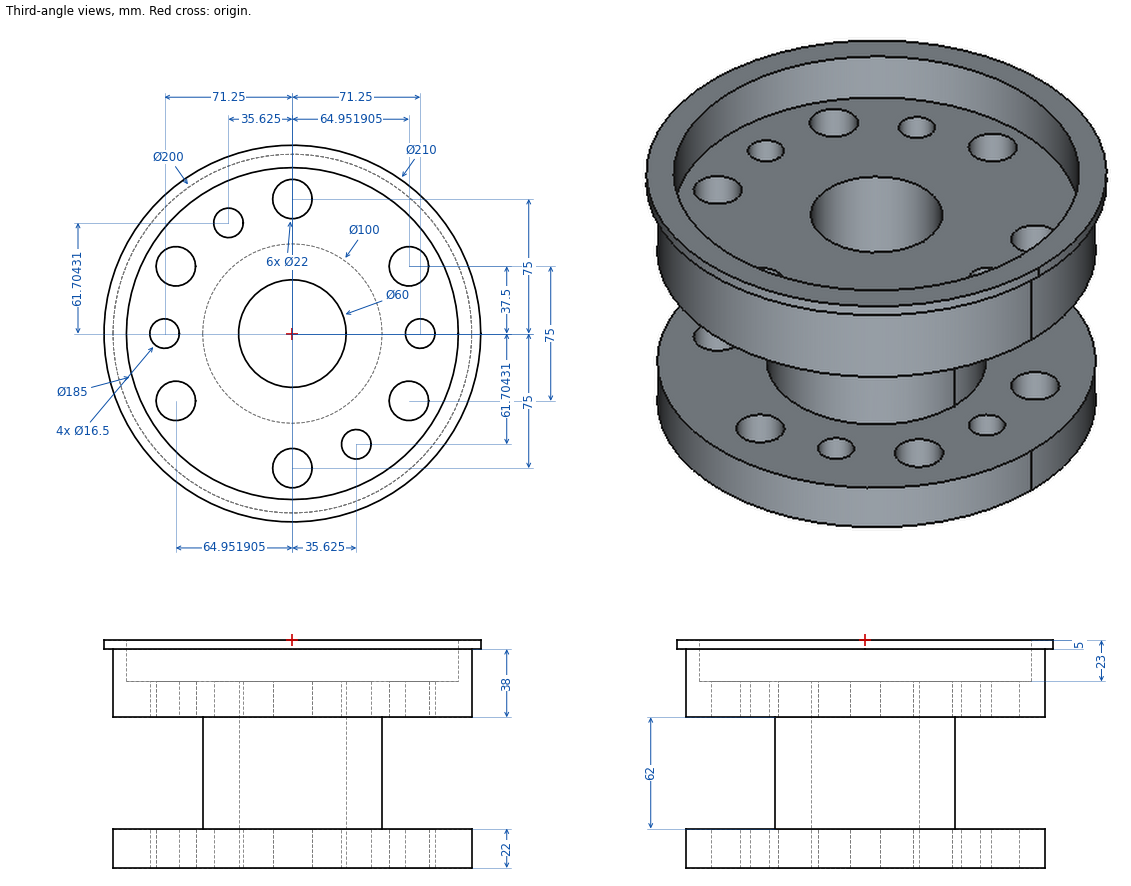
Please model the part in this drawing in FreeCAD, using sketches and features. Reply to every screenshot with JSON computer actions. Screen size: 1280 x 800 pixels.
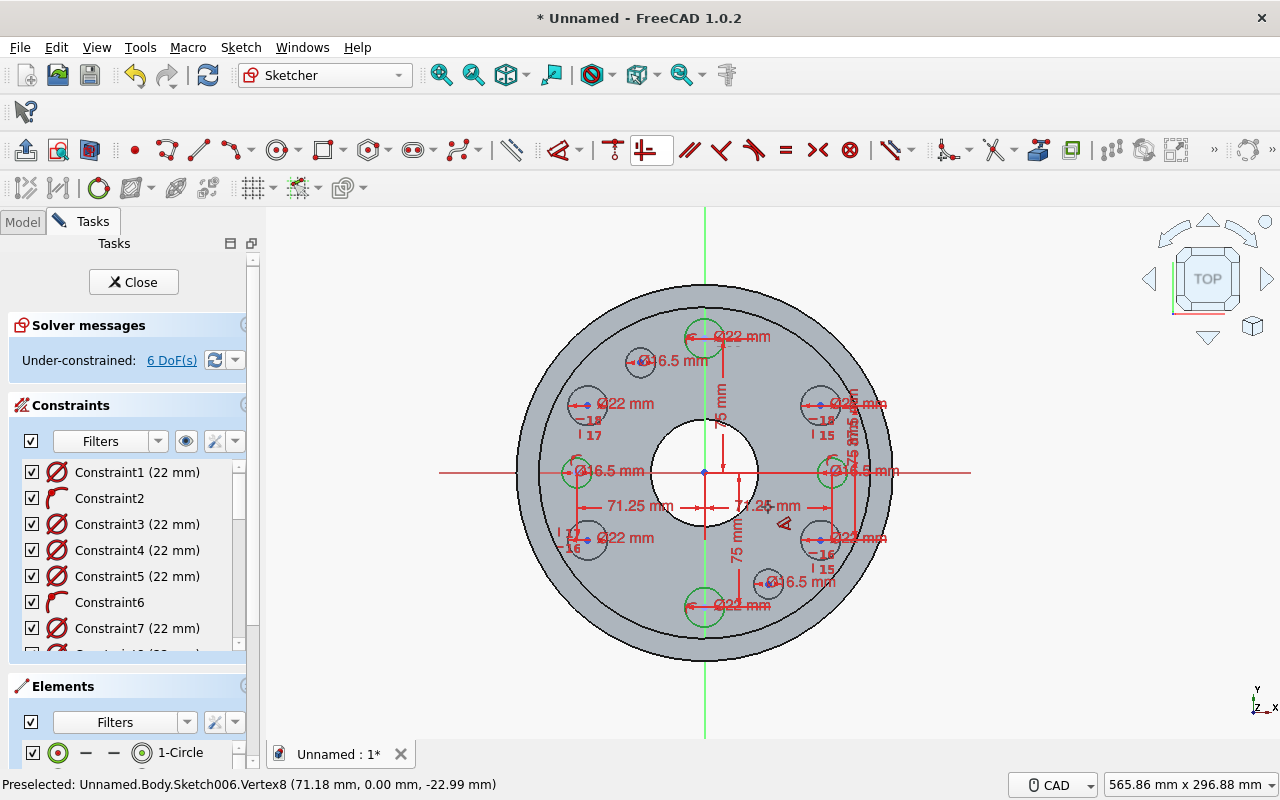
{"action": "left_click", "coordinate": [769, 584]}
{"action": "left_click", "coordinate": [737, 618]}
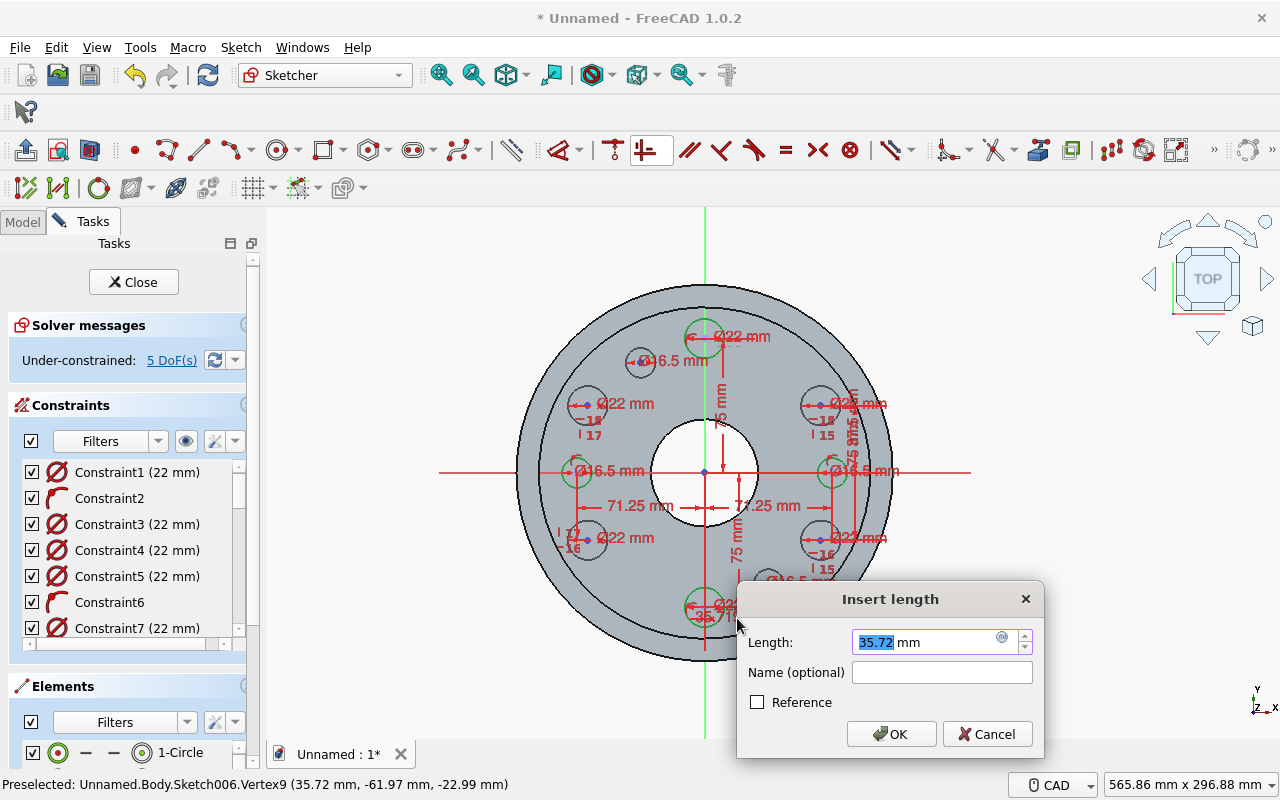
{"action": "type", "text": "35.625"}
{"action": "key", "text": "Return"}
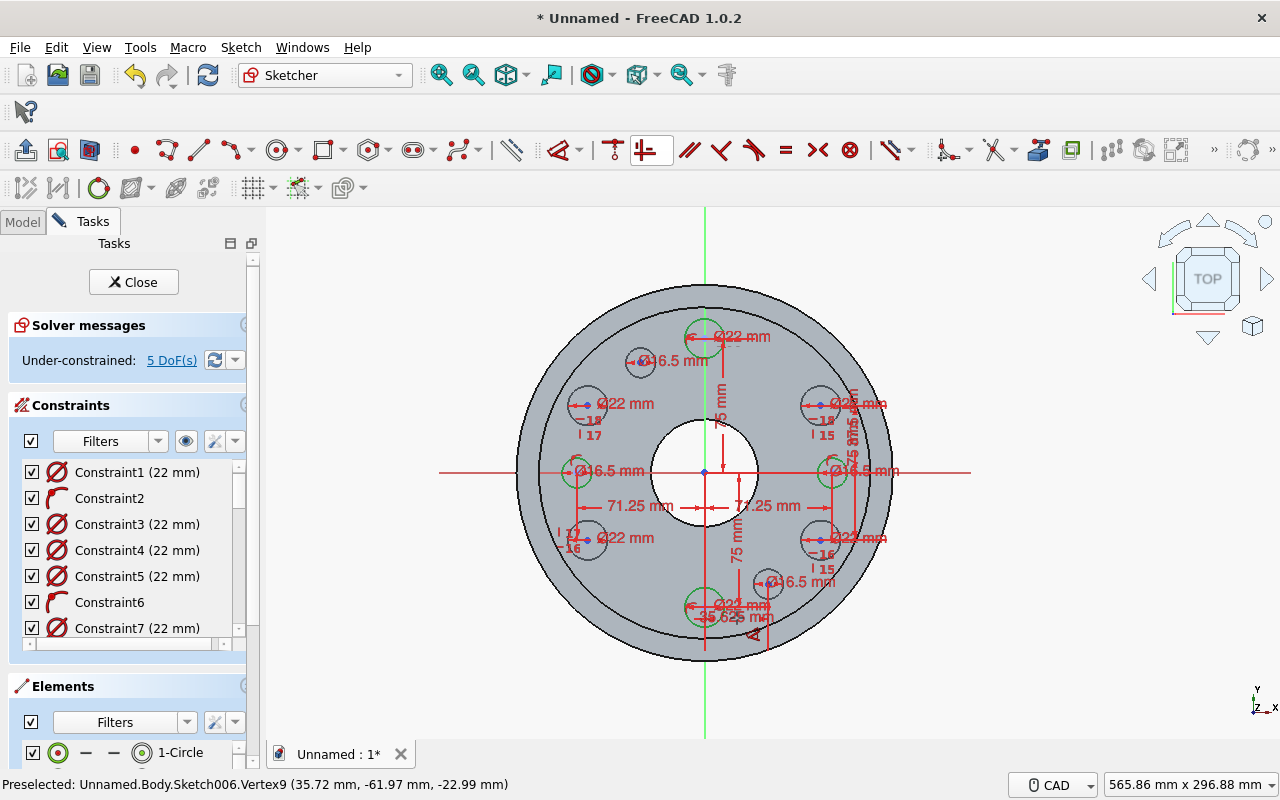
{"action": "left_click", "coordinate": [641, 363]}
{"action": "left_click", "coordinate": [673, 329]}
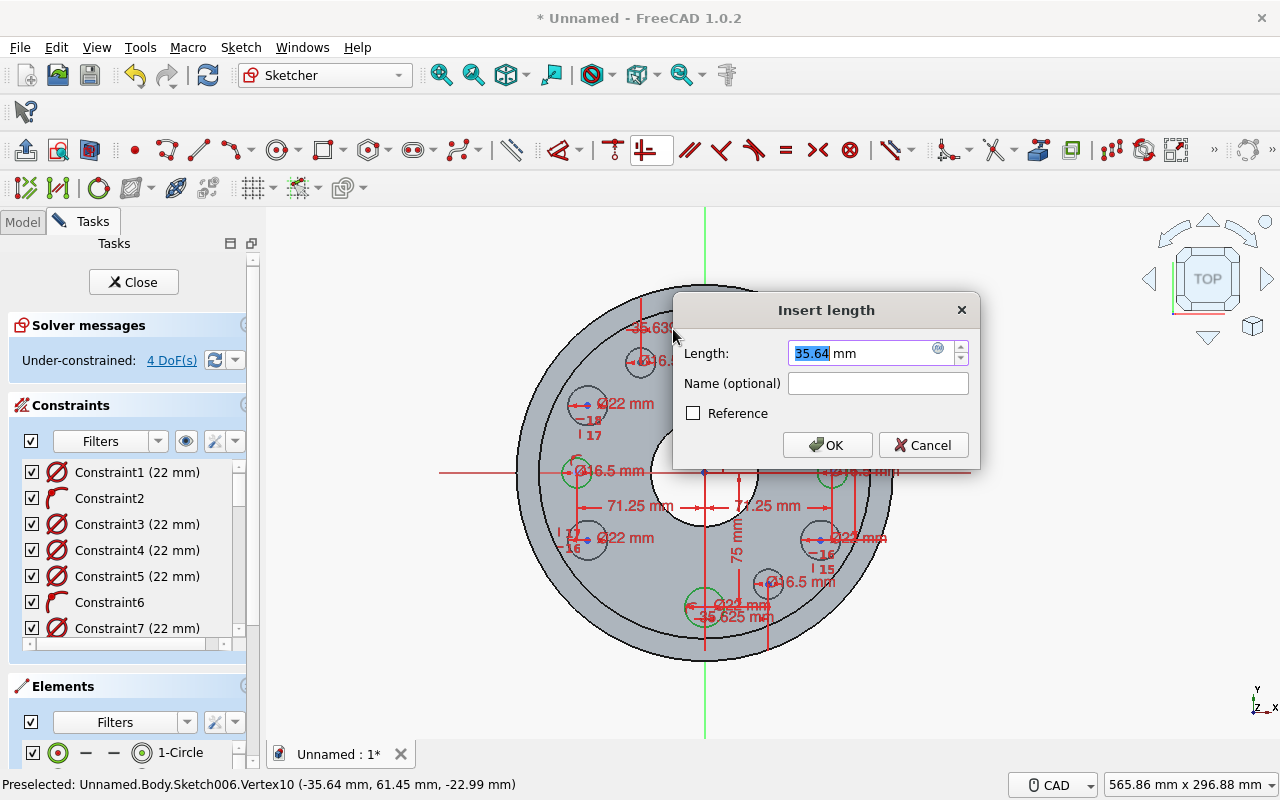
{"action": "type", "text": "35.625"}
{"action": "key", "text": "Return"}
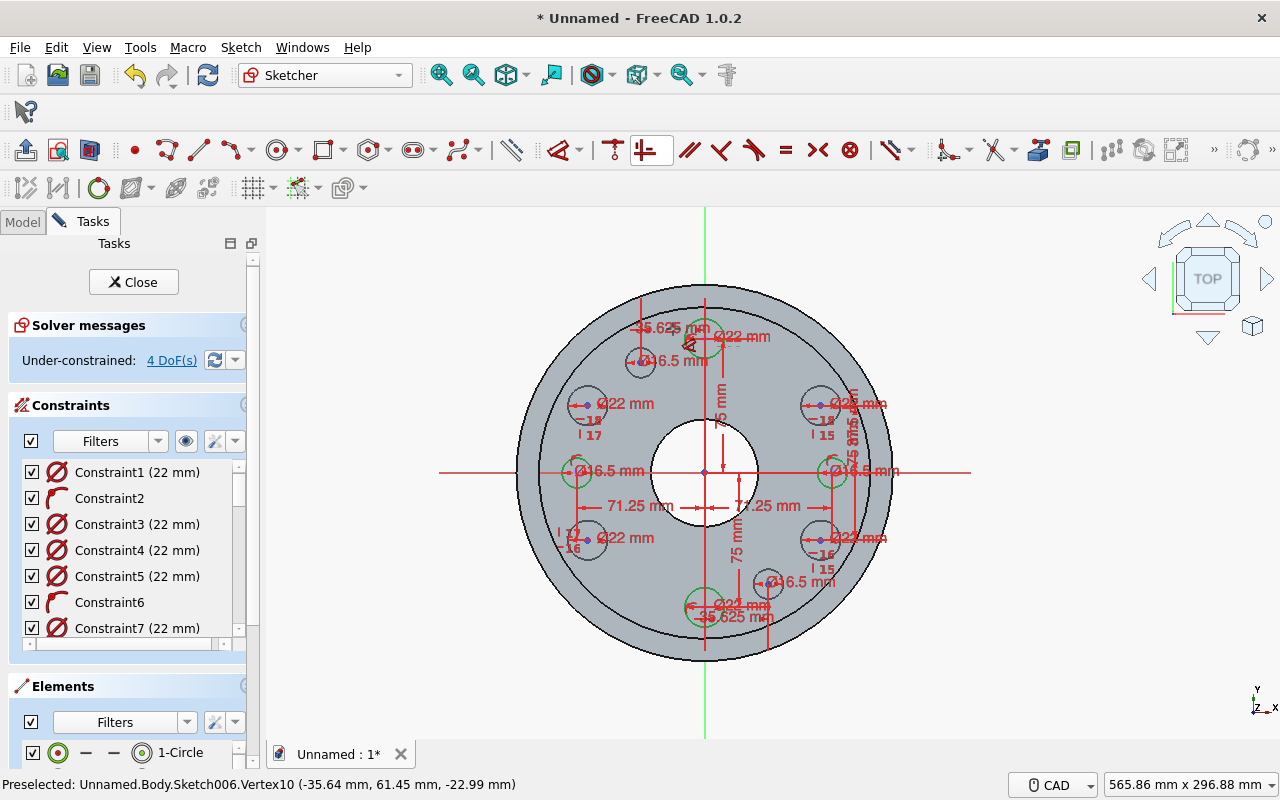
{"action": "left_click", "coordinate": [768, 584]}
{"action": "left_click", "coordinate": [802, 567]}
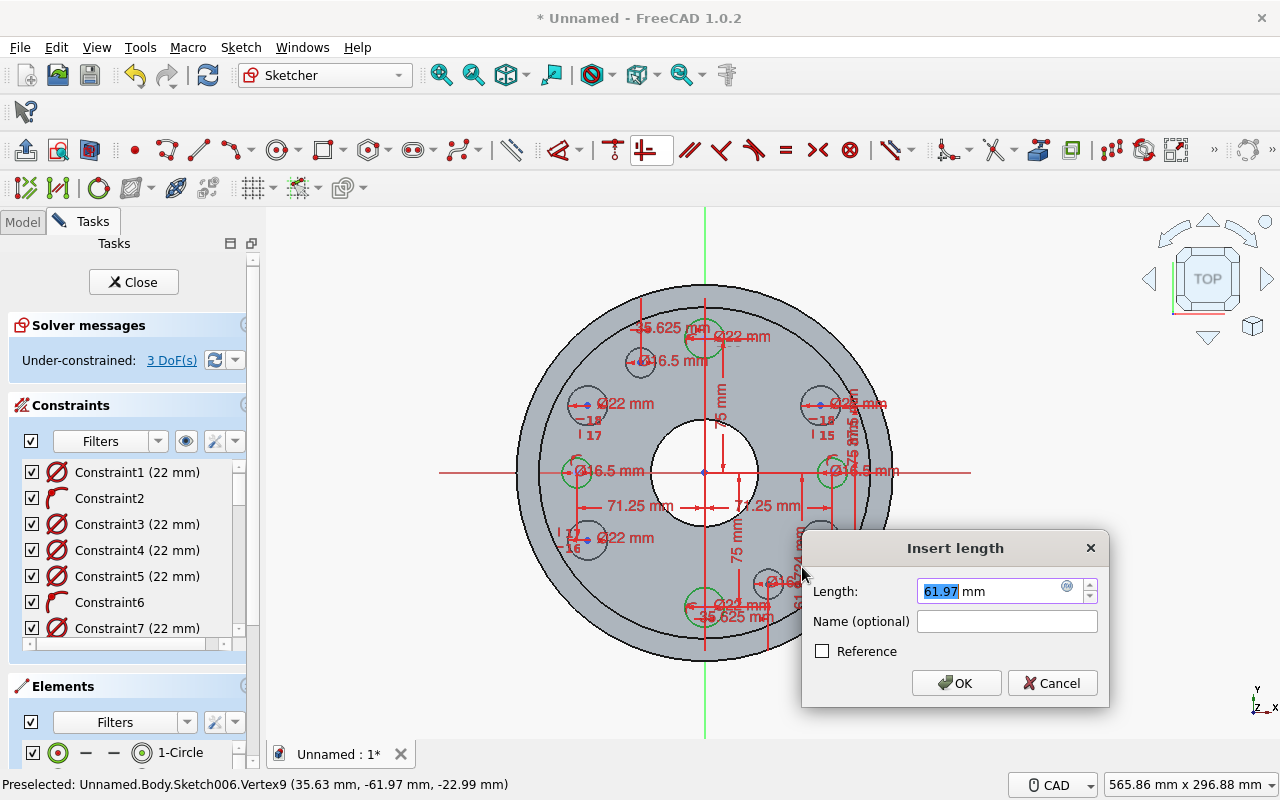
{"action": "type", "text": "61.70431"}
{"action": "key", "text": "Return"}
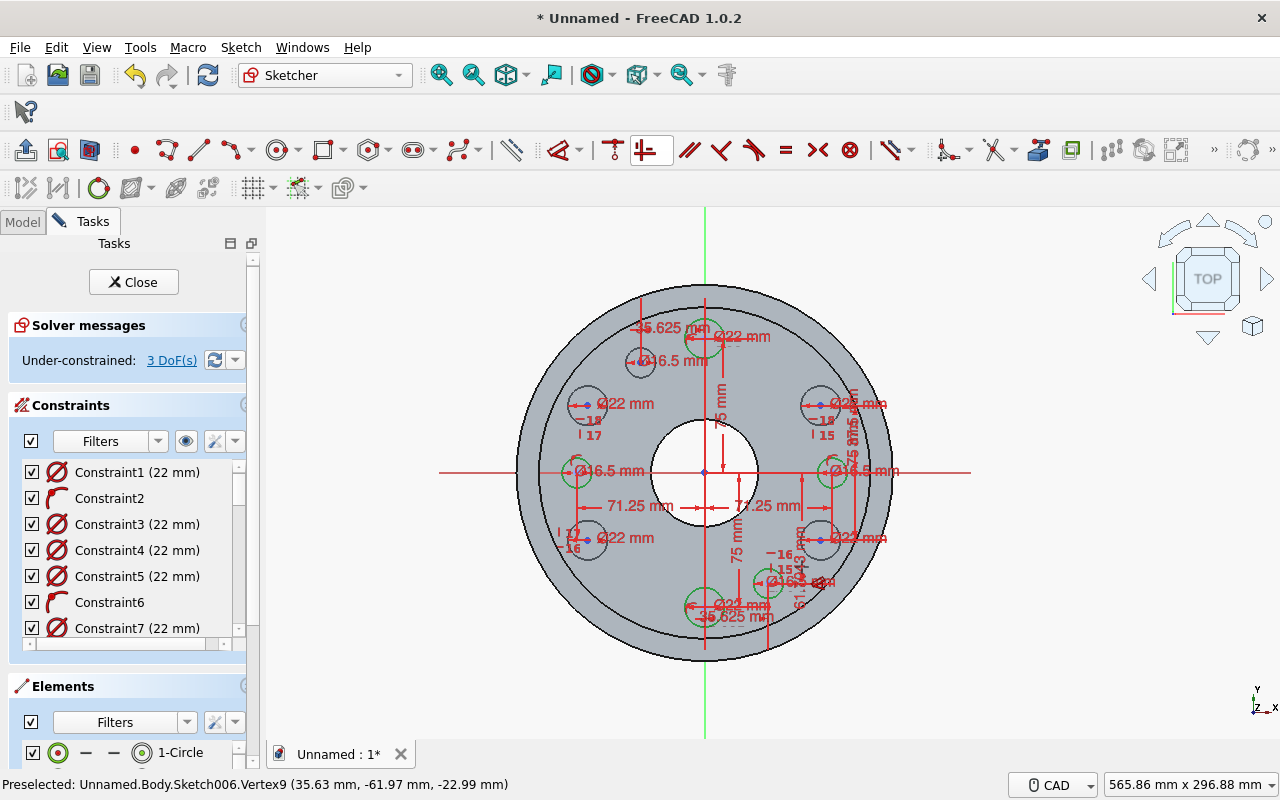
{"action": "left_click", "coordinate": [641, 363]}
{"action": "left_click", "coordinate": [607, 443]}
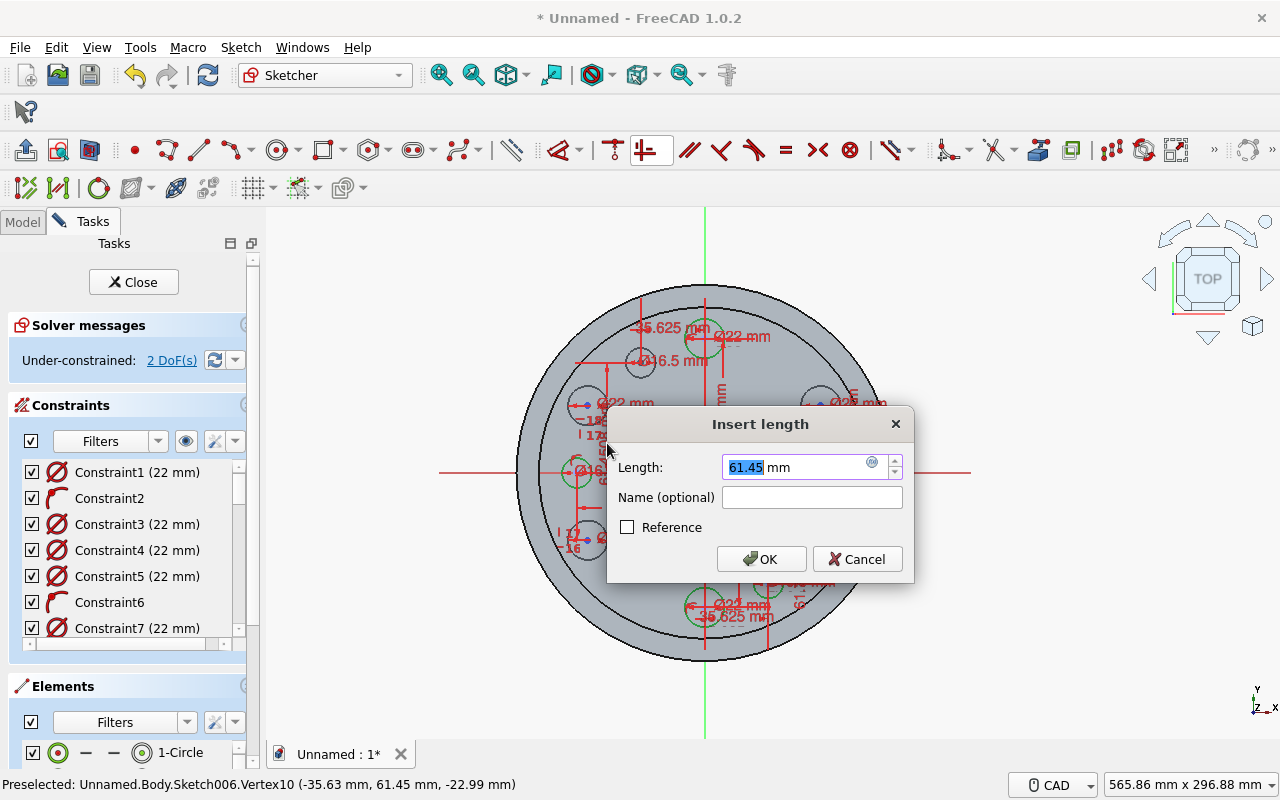
{"action": "type", "text": "61.70431"}
{"action": "key", "text": "Return"}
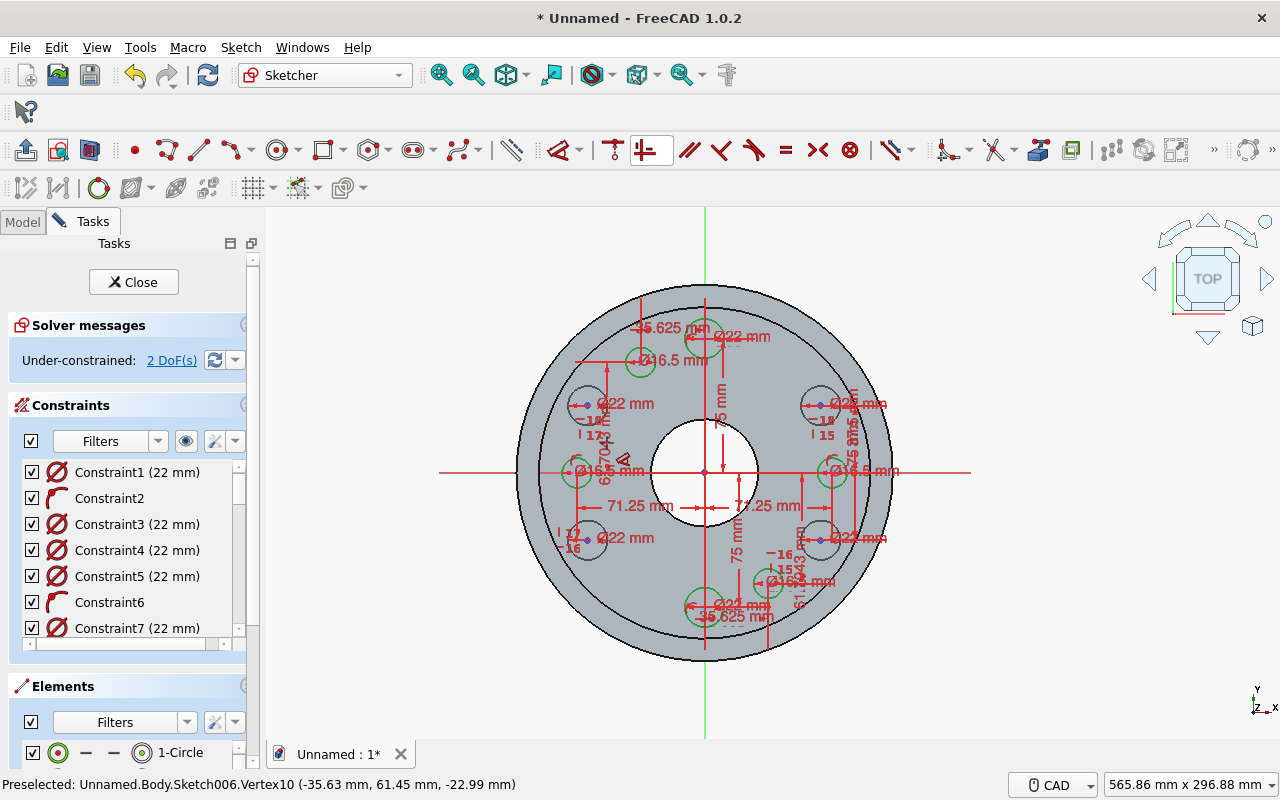
{"action": "left_click", "coordinate": [821, 406]}
{"action": "left_click", "coordinate": [763, 372]}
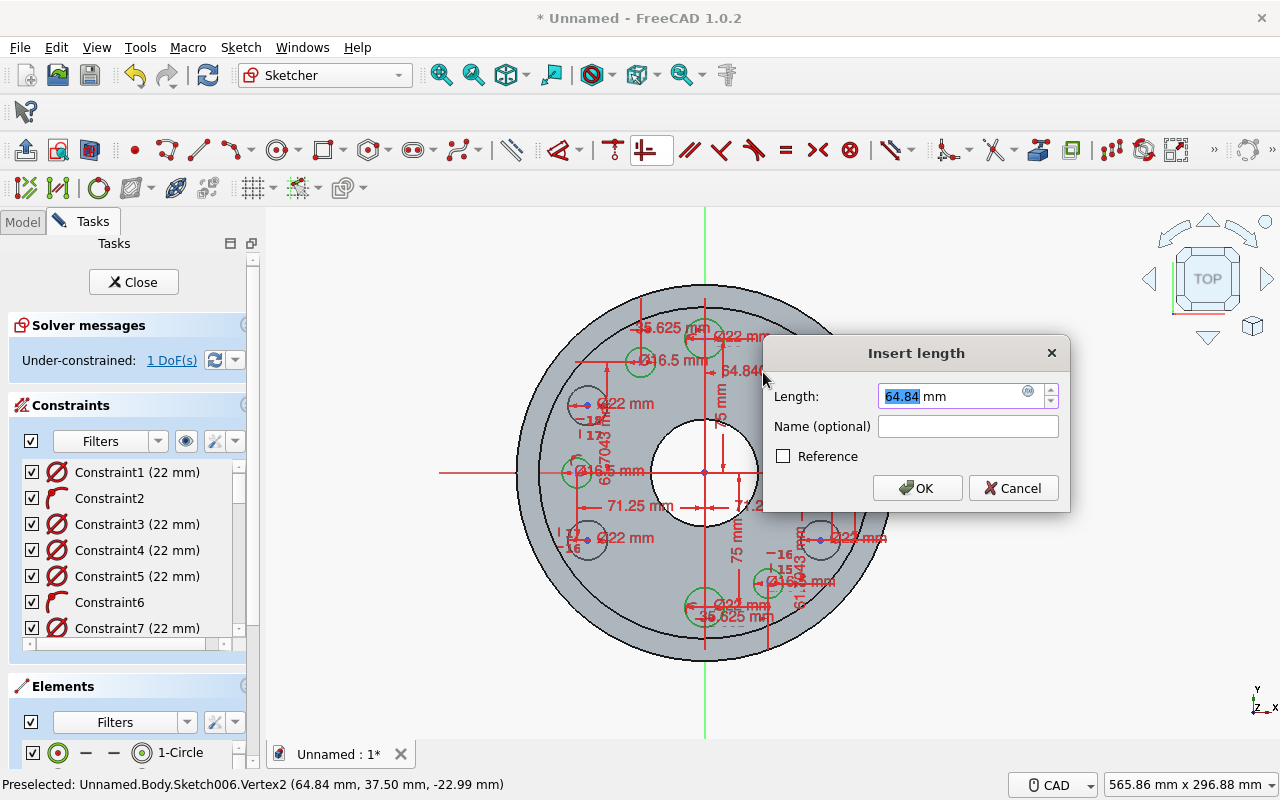
{"action": "type", "text": "64.951905"}
{"action": "key", "text": "Return"}